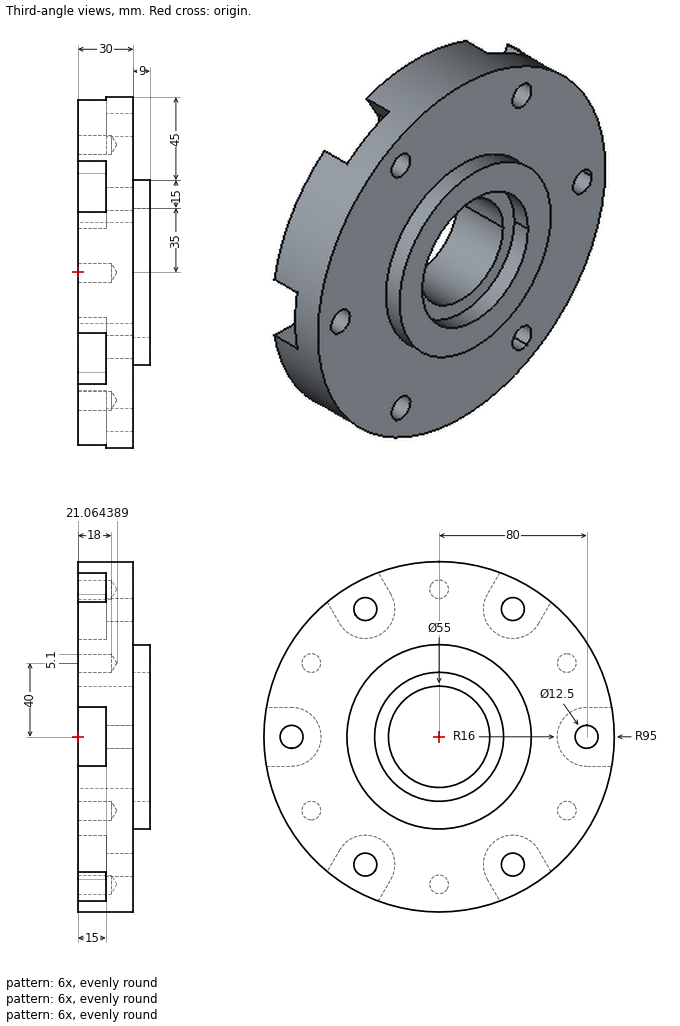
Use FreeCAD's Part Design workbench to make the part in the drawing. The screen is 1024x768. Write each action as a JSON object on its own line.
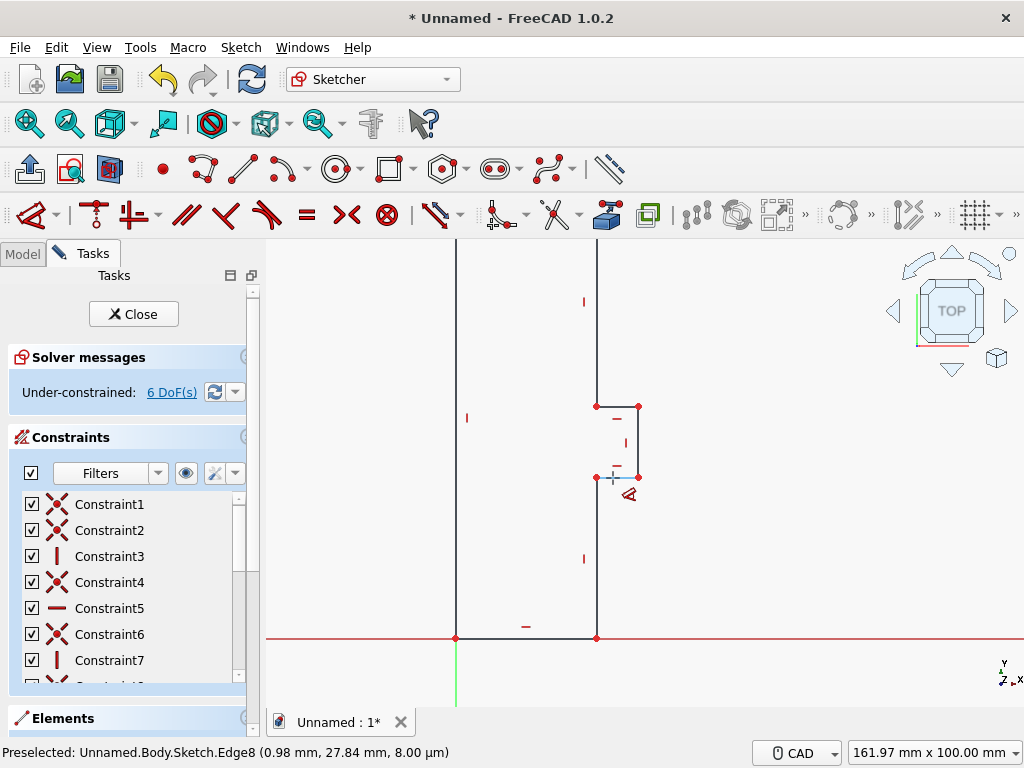
{"action": "left_click", "coordinate": [613, 478]}
{"action": "left_click", "coordinate": [617, 512]}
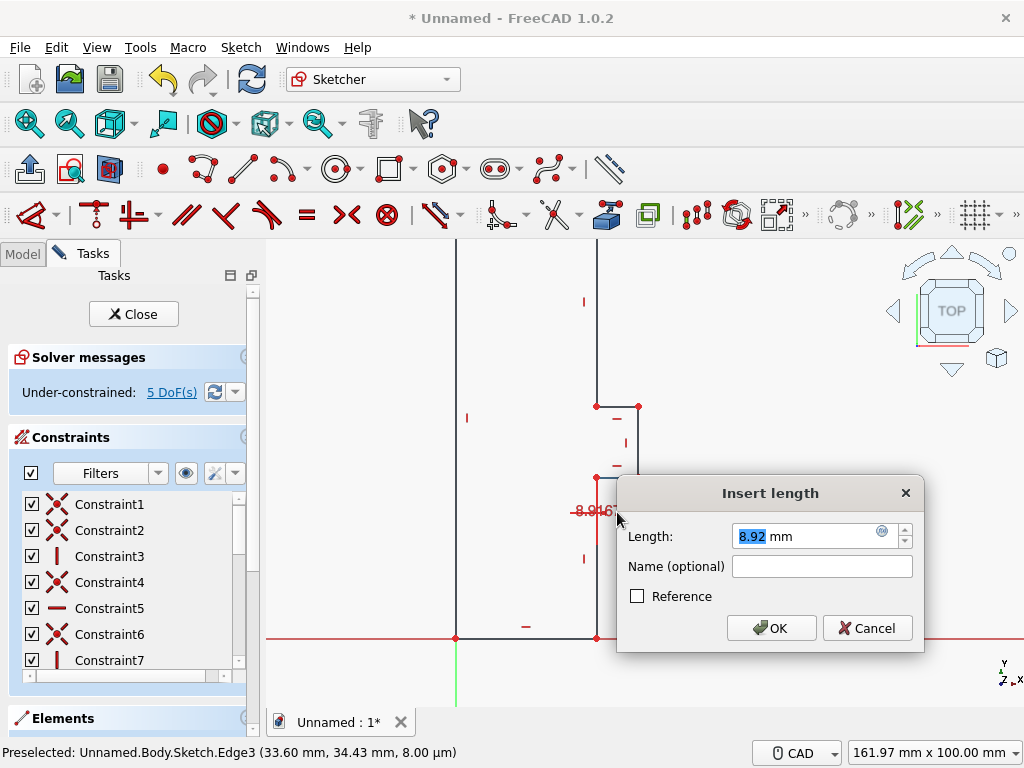
{"action": "type", "text": "9"}
{"action": "key", "text": "Return"}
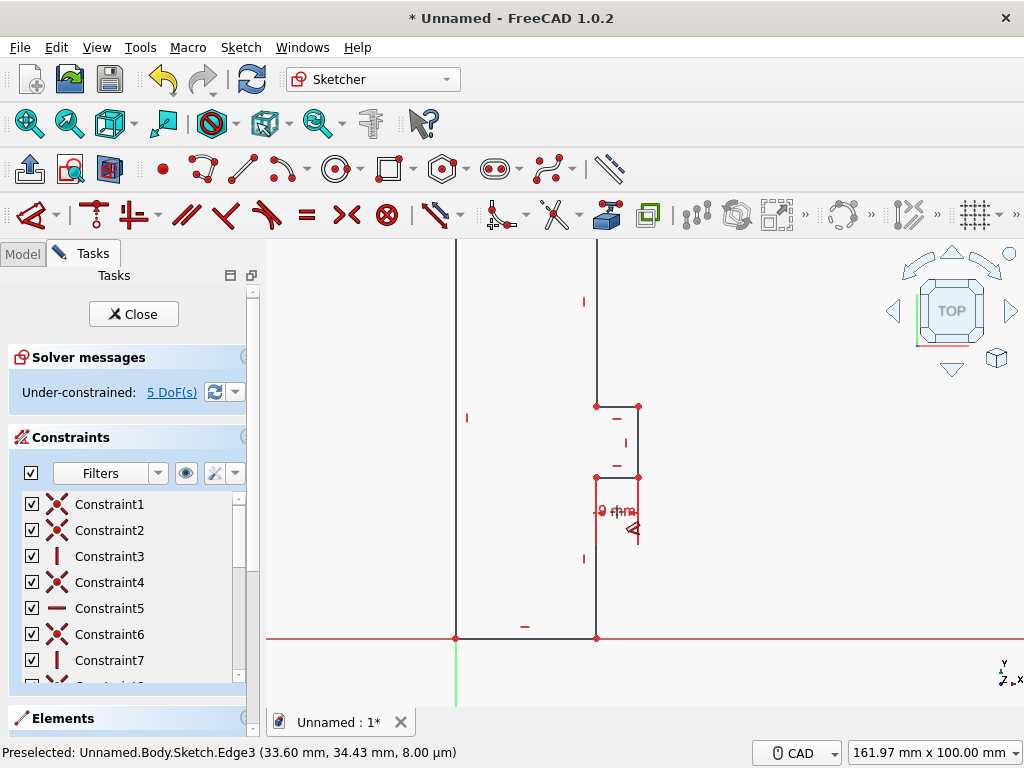
{"action": "left_click", "coordinate": [626, 407]}
{"action": "left_click", "coordinate": [617, 373]}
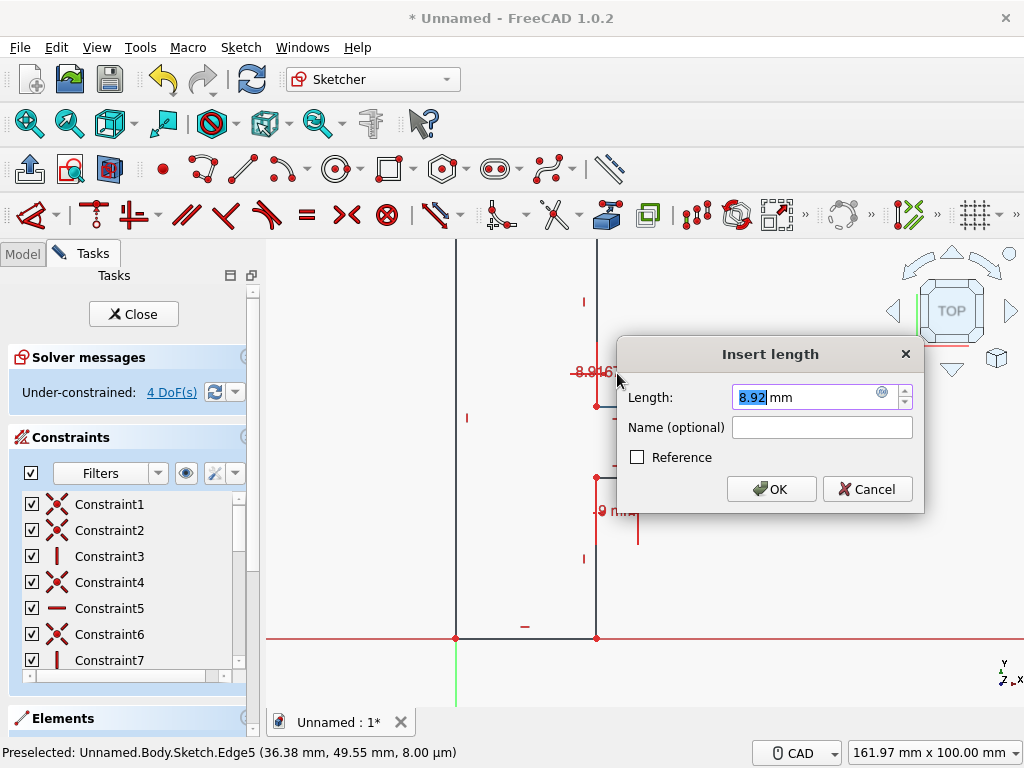
{"action": "type", "text": "9"}
{"action": "key", "text": "Return"}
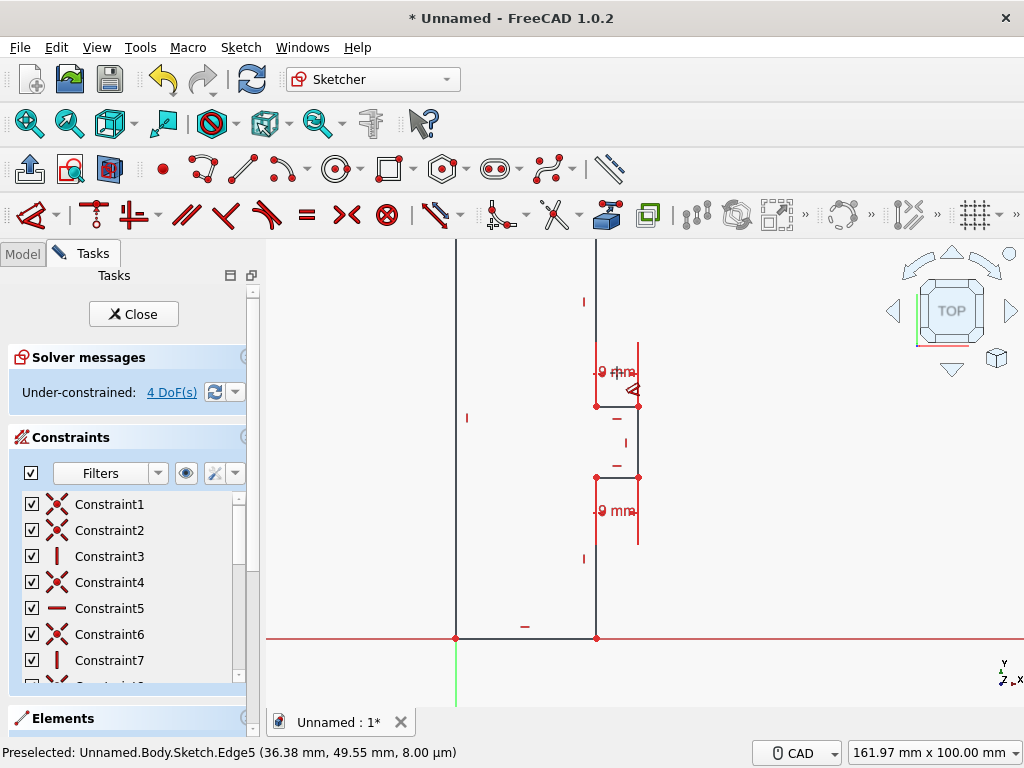
{"action": "left_click", "coordinate": [498, 639]}
{"action": "left_click", "coordinate": [526, 673]}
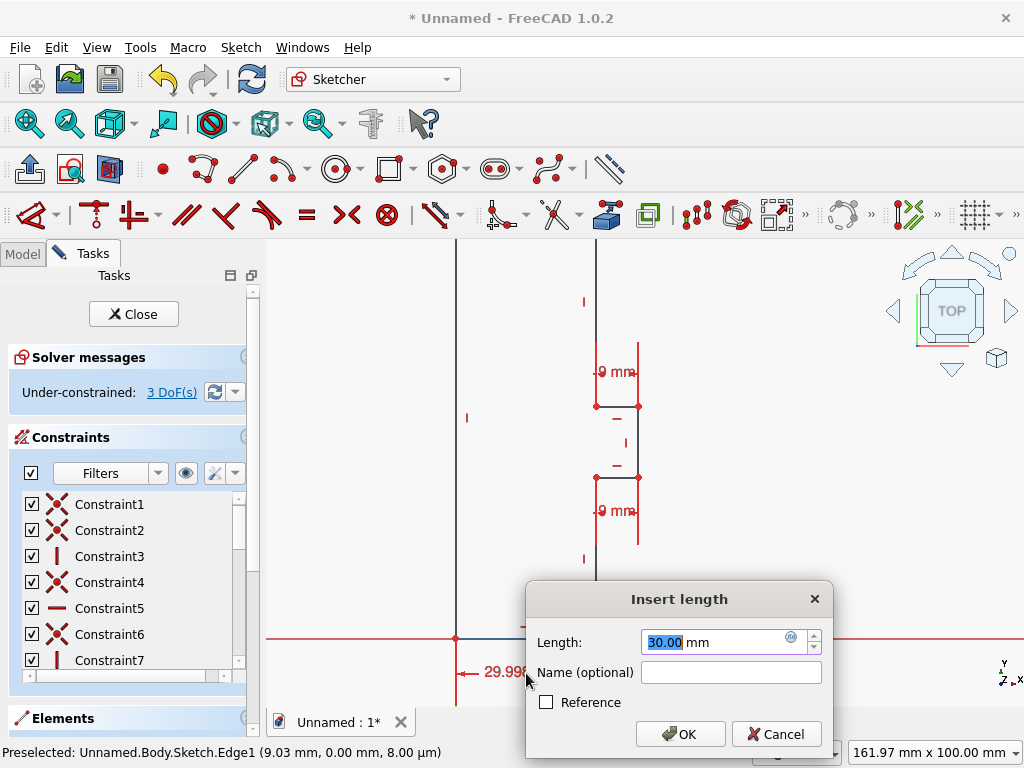
{"action": "type", "text": "30"}
{"action": "key", "text": "Return"}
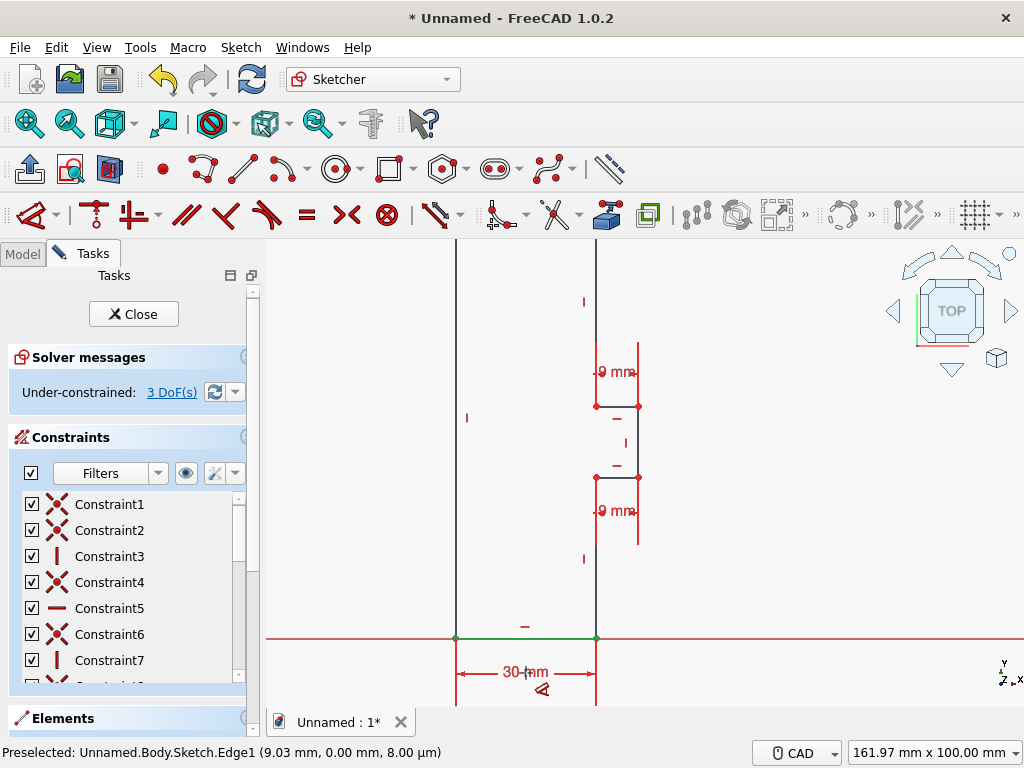
{"action": "left_click", "coordinate": [596, 590]}
{"action": "left_click", "coordinate": [630, 558]}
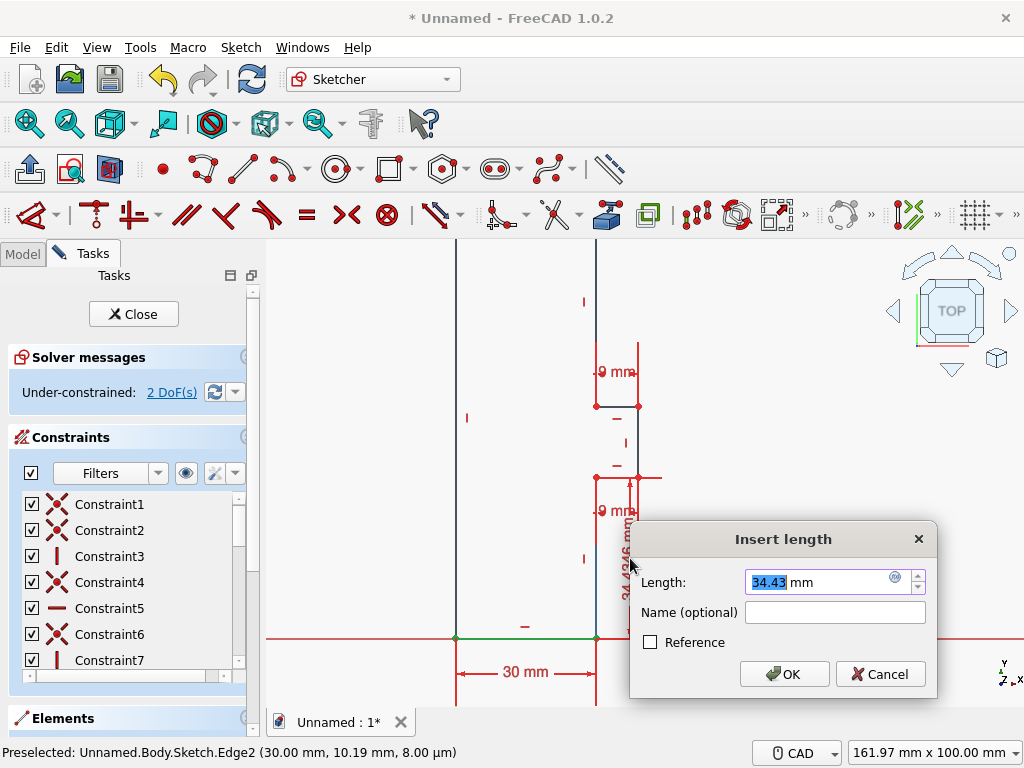
{"action": "type", "text": "35"}
{"action": "key", "text": "Return"}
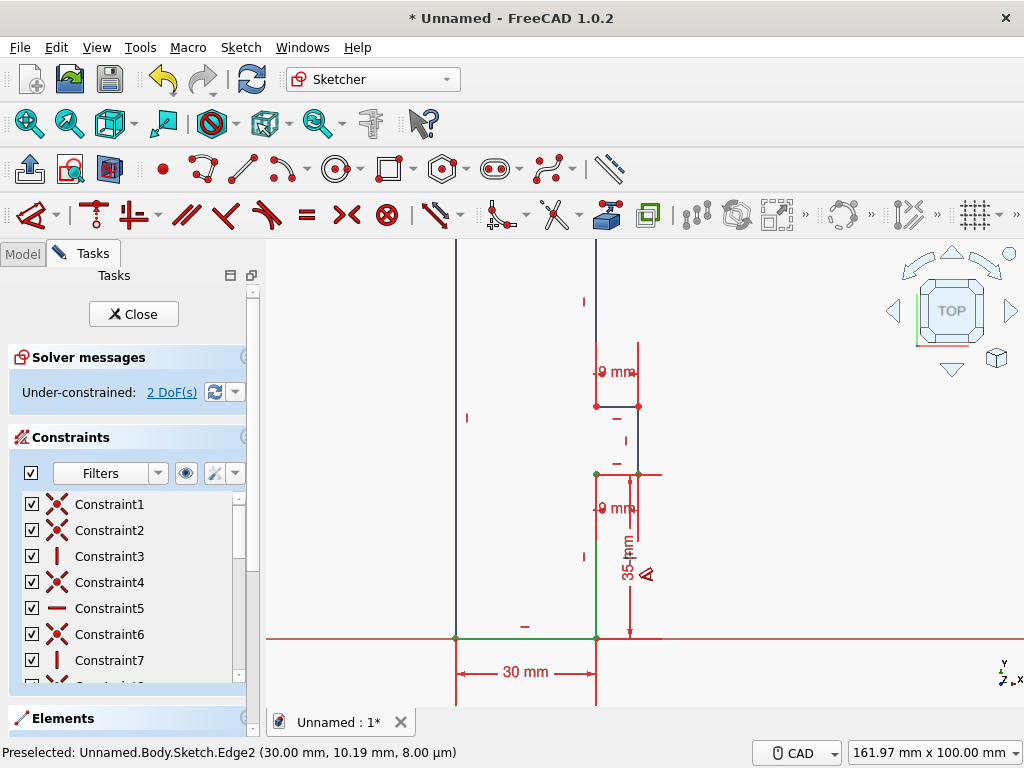
{"action": "left_click", "coordinate": [638, 454]}
{"action": "left_click", "coordinate": [672, 441]}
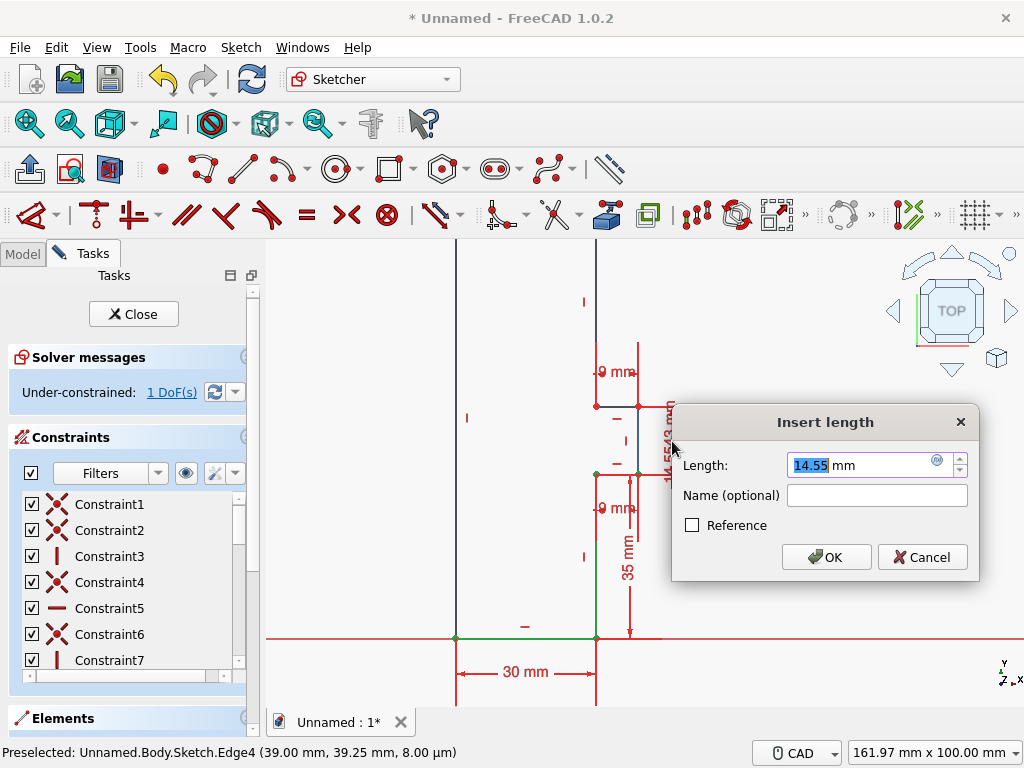
{"action": "type", "text": "15"}
{"action": "key", "text": "Return"}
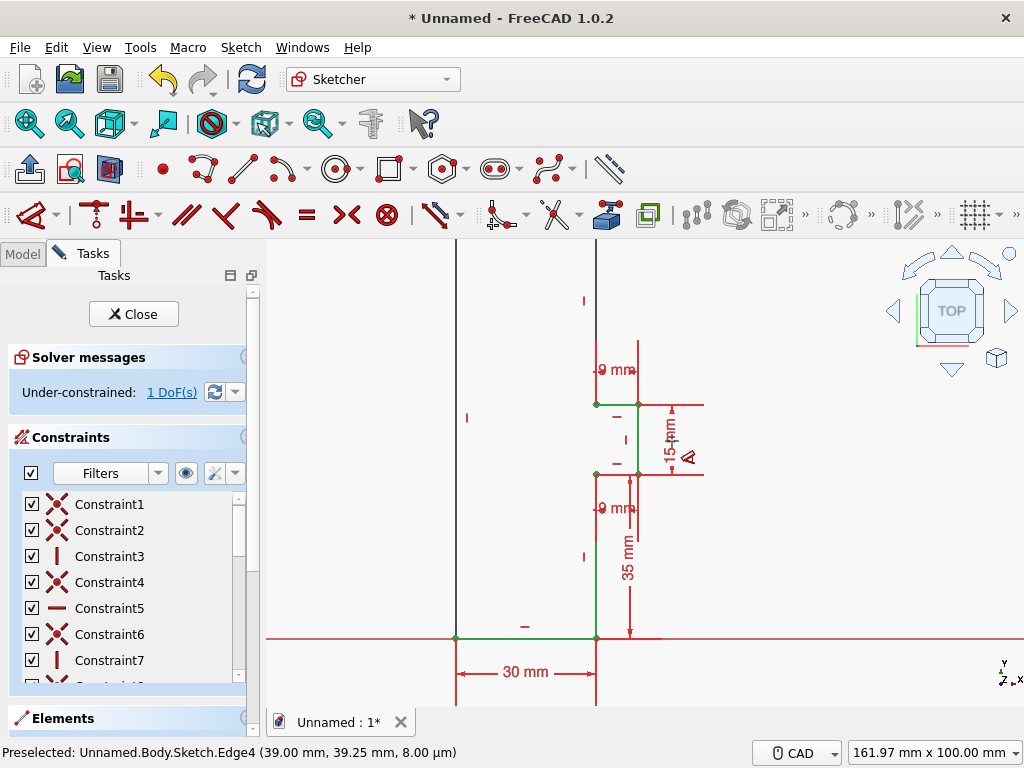
{"action": "left_click", "coordinate": [596, 342]}
{"action": "left_click", "coordinate": [630, 336]}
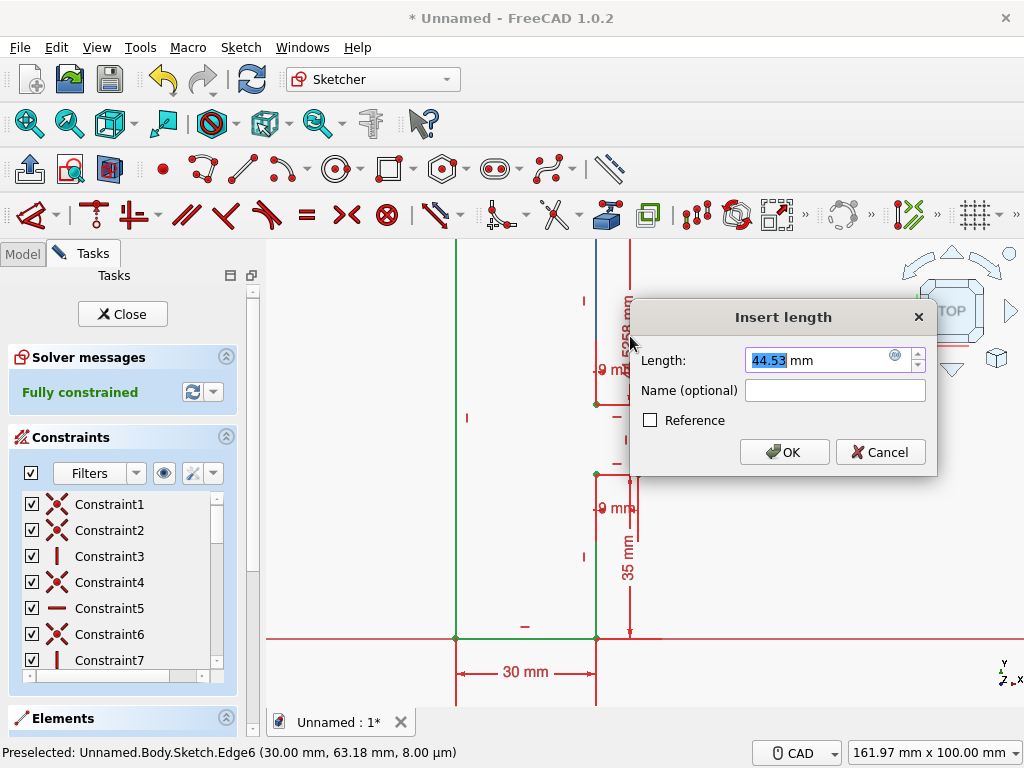
{"action": "type", "text": "45"}
{"action": "key", "text": "Return"}
{"action": "key", "text": "Escape"}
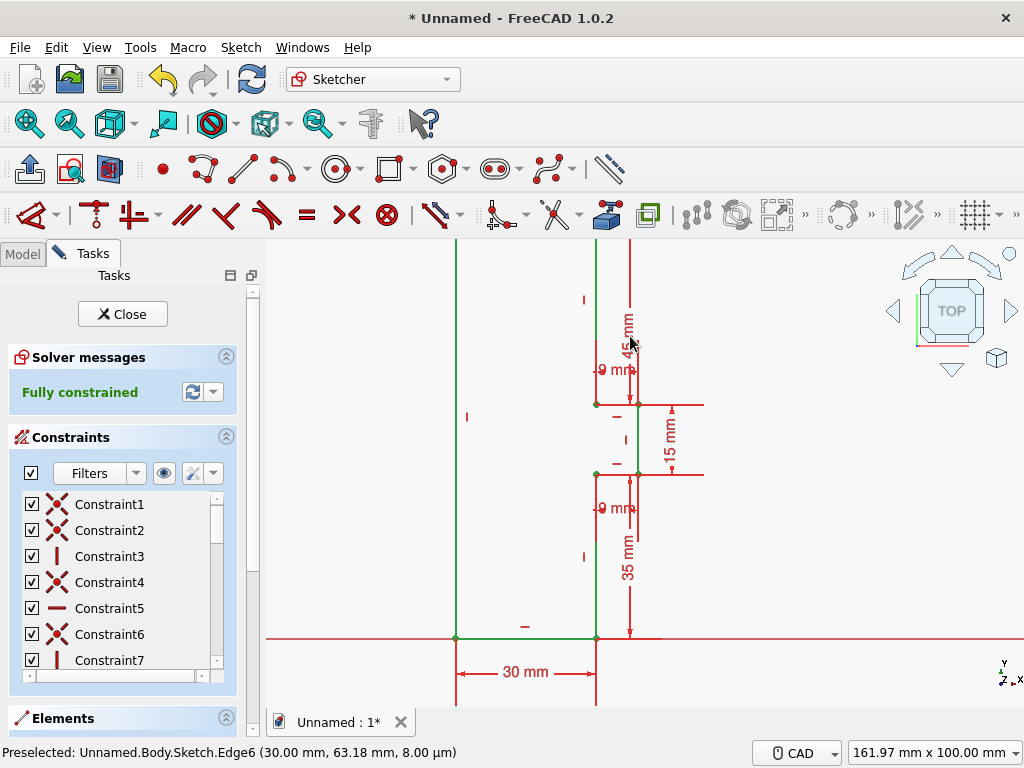
{"action": "left_click", "coordinate": [123, 314]}